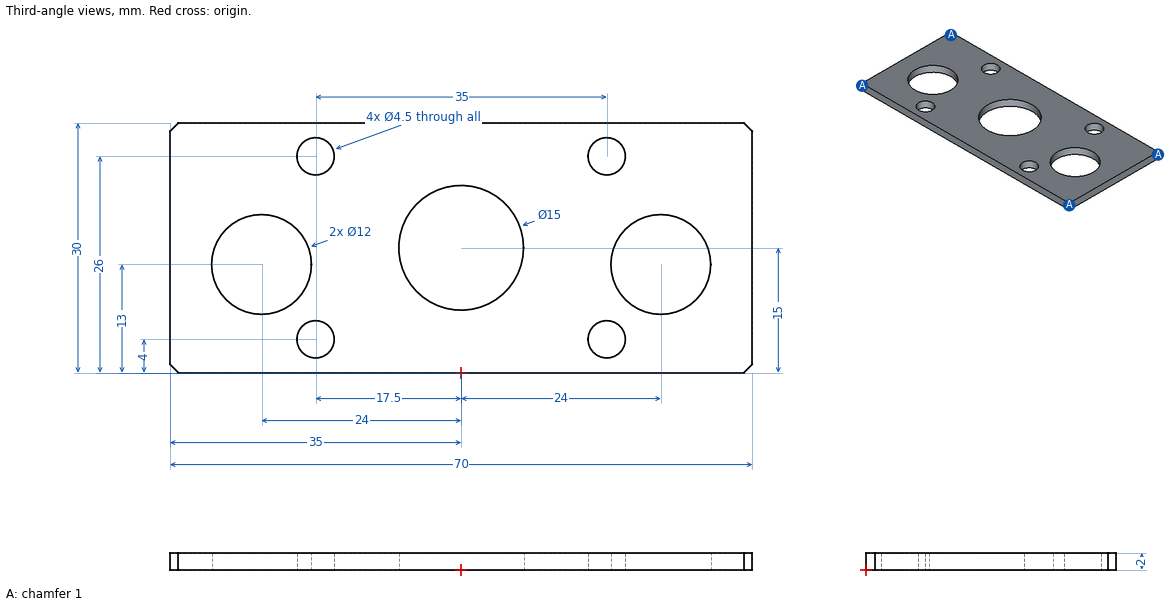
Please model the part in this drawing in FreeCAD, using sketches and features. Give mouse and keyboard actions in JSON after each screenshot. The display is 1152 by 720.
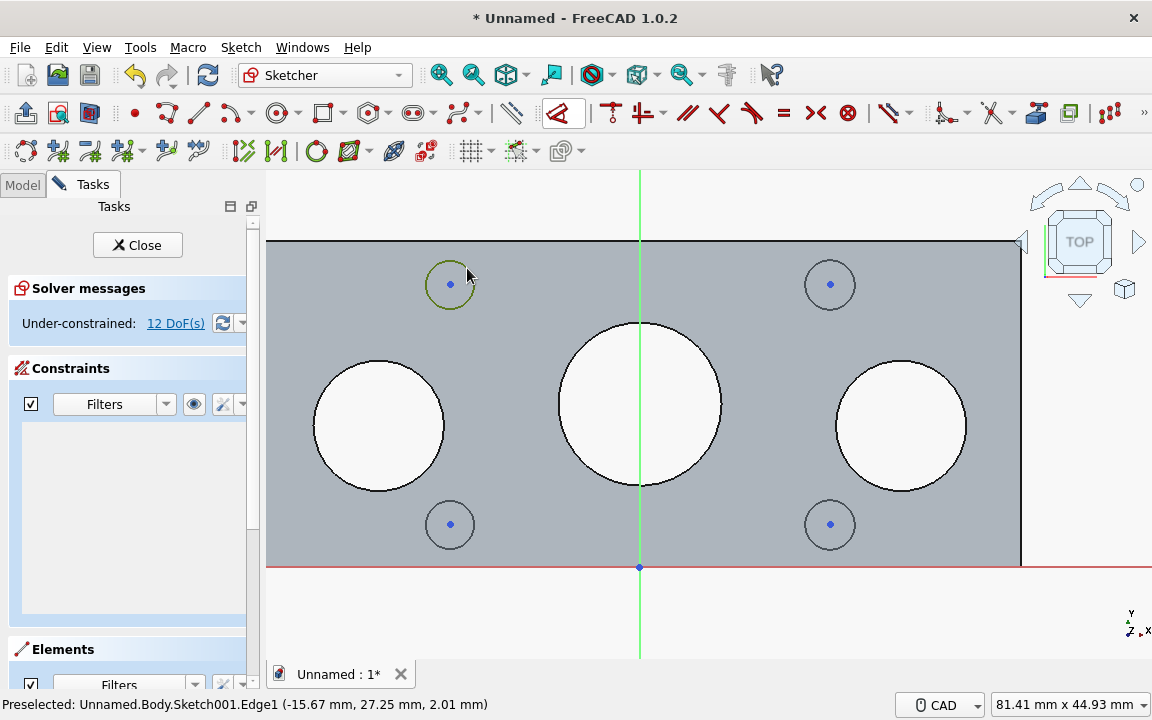
{"action": "left_click", "coordinate": [847, 267]}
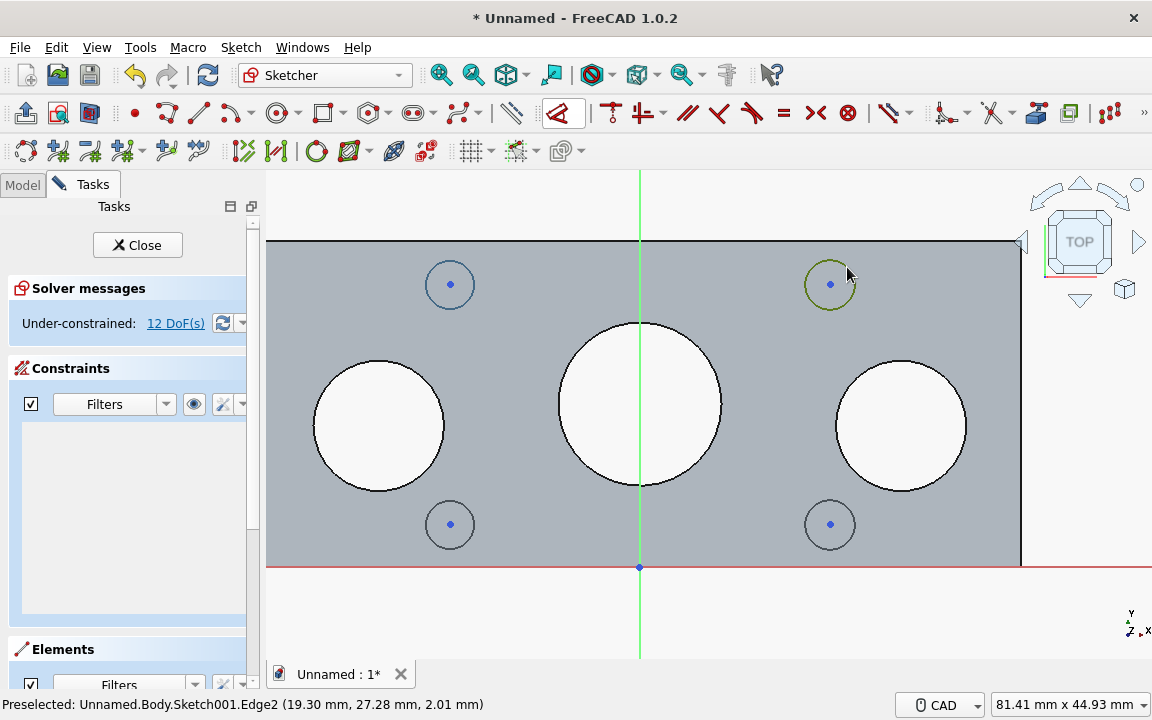
{"action": "left_click", "coordinate": [467, 508]}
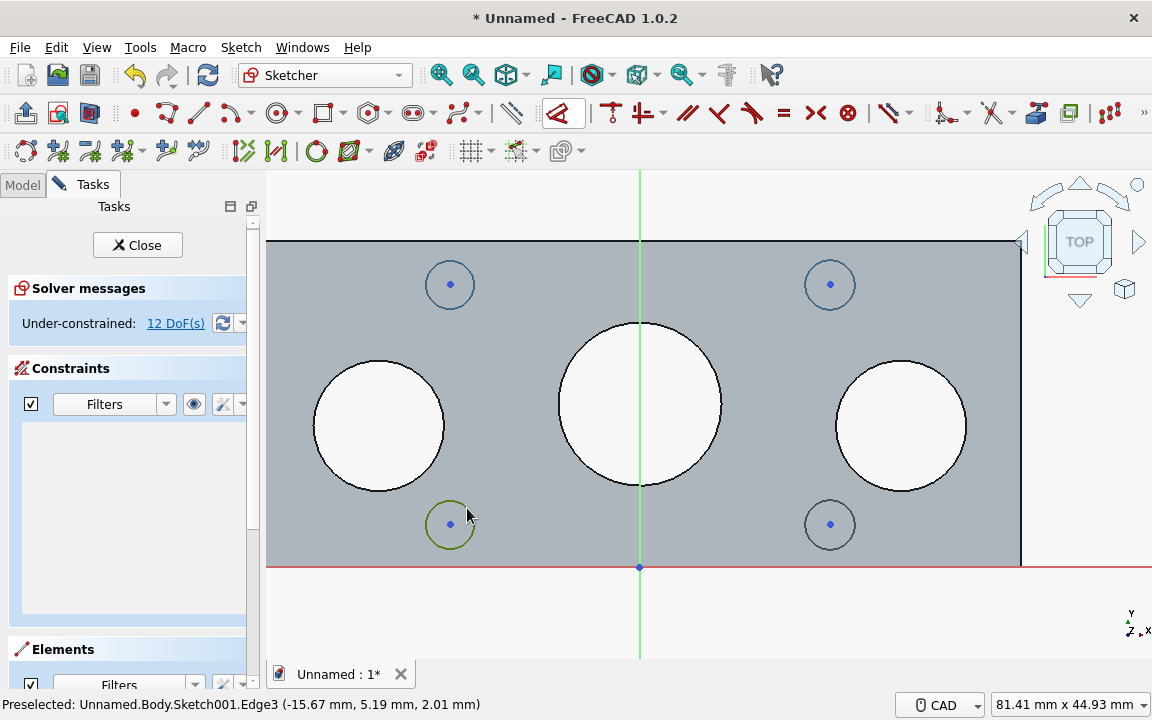
{"action": "left_click", "coordinate": [847, 507]}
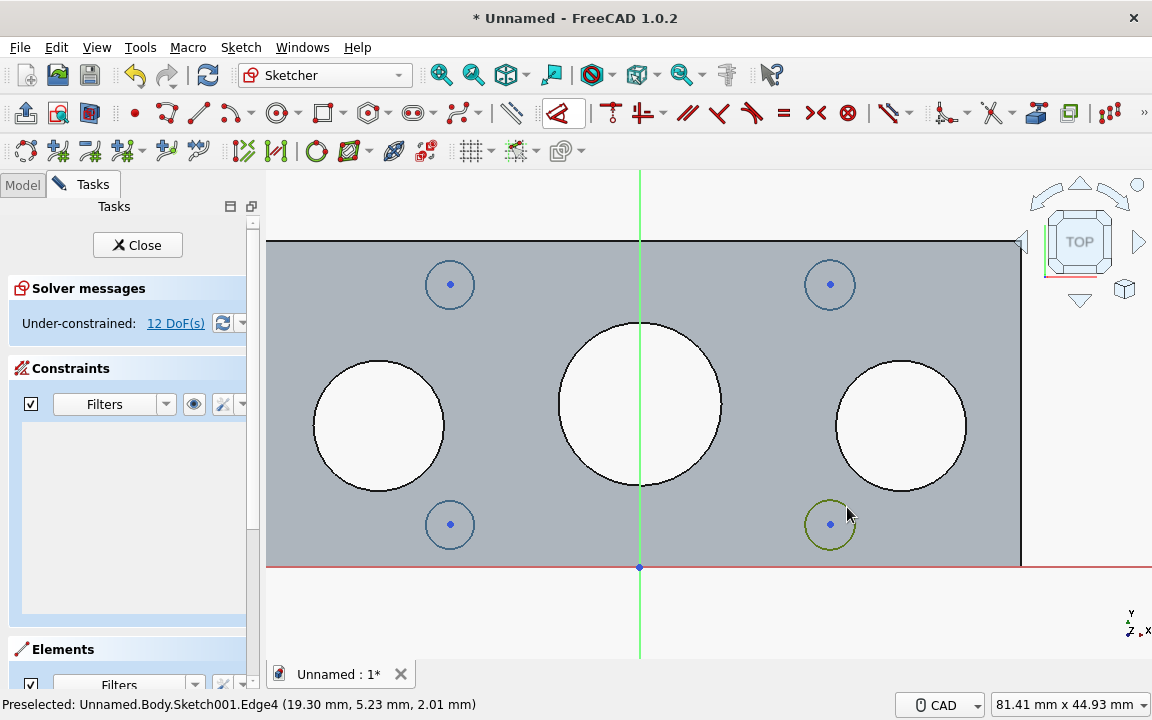
{"action": "left_click", "coordinate": [784, 114]}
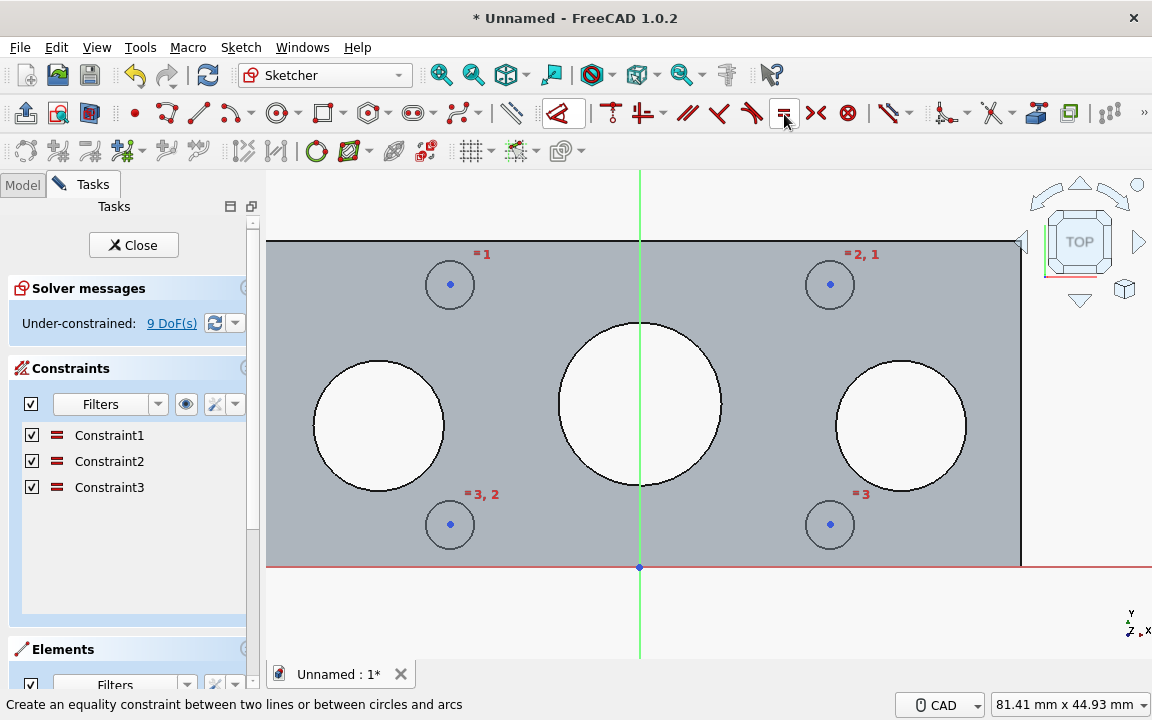
{"action": "left_click", "coordinate": [450, 285]}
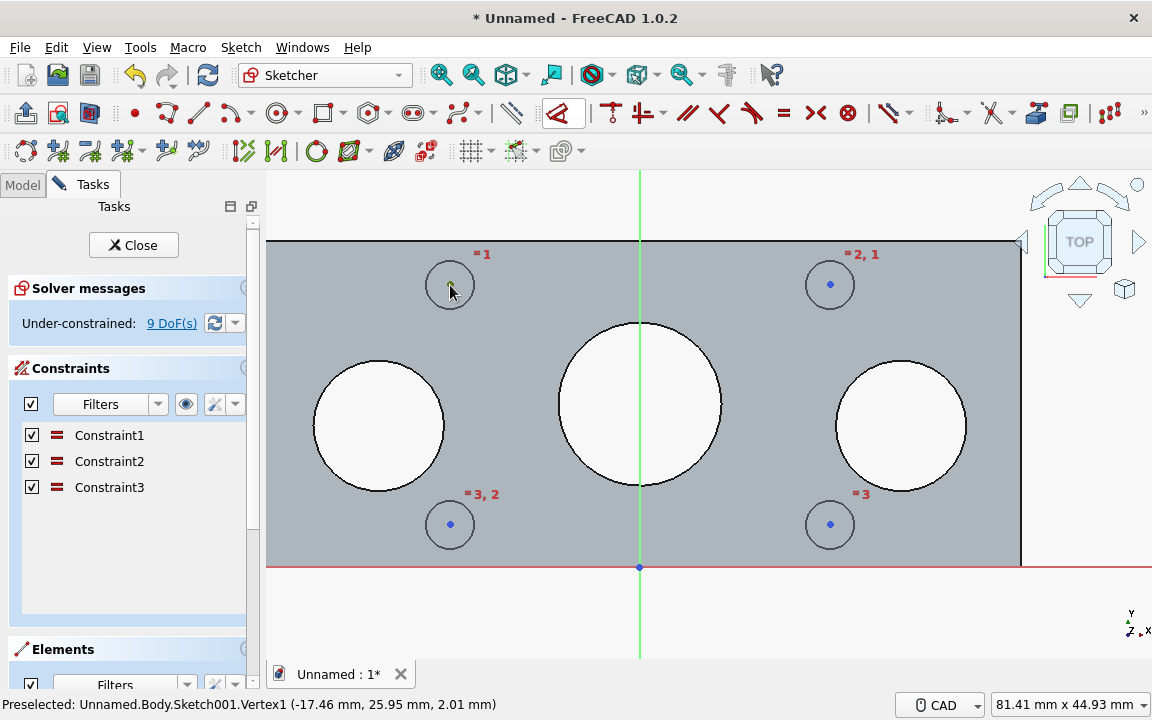
{"action": "left_click", "coordinate": [830, 285]}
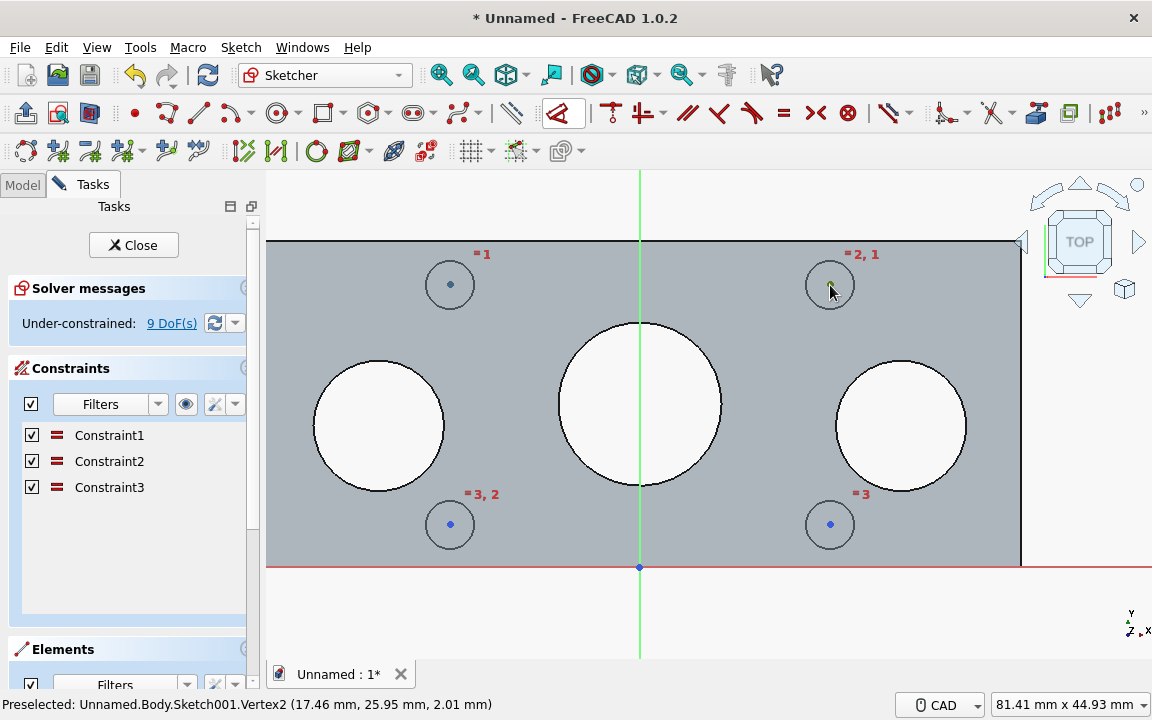
{"action": "left_click", "coordinate": [666, 114]}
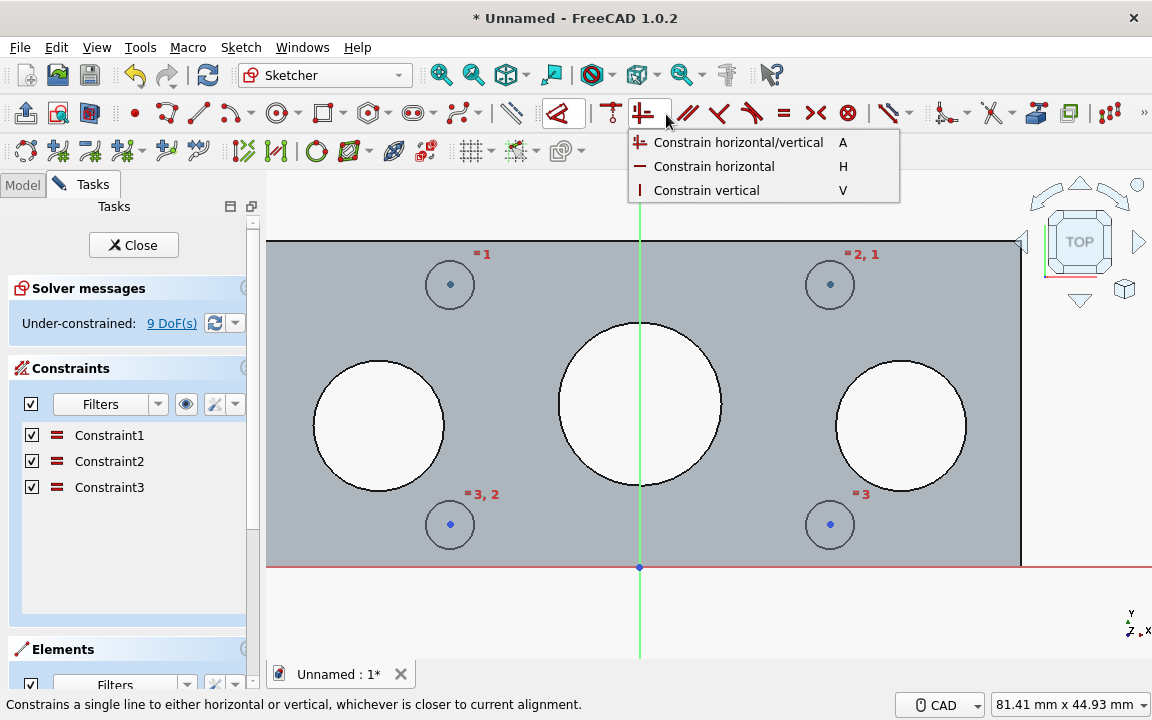
{"action": "left_click", "coordinate": [764, 166]}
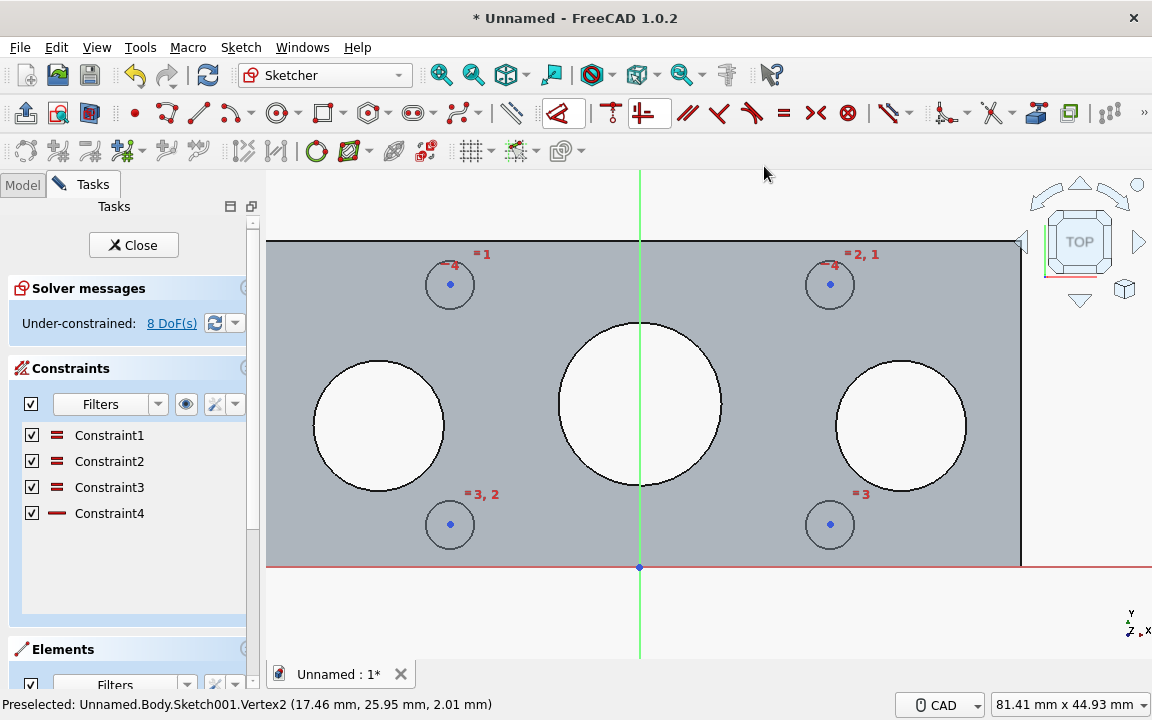
{"action": "left_click", "coordinate": [450, 285]}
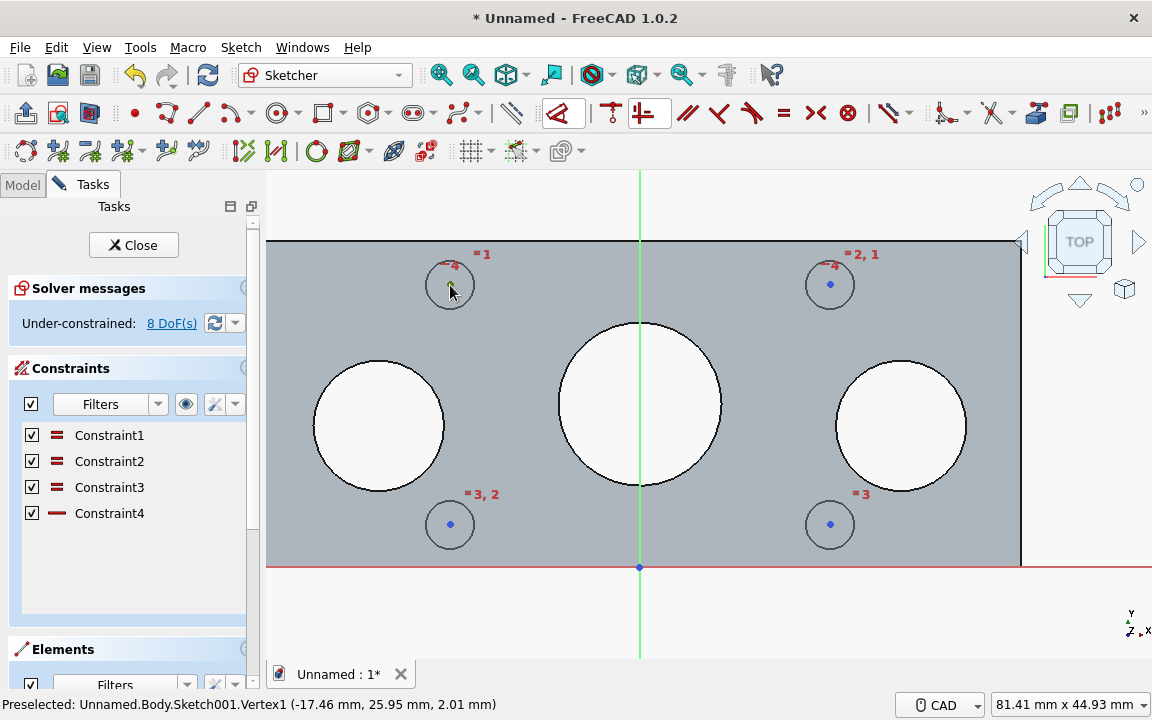
{"action": "left_click", "coordinate": [450, 525]}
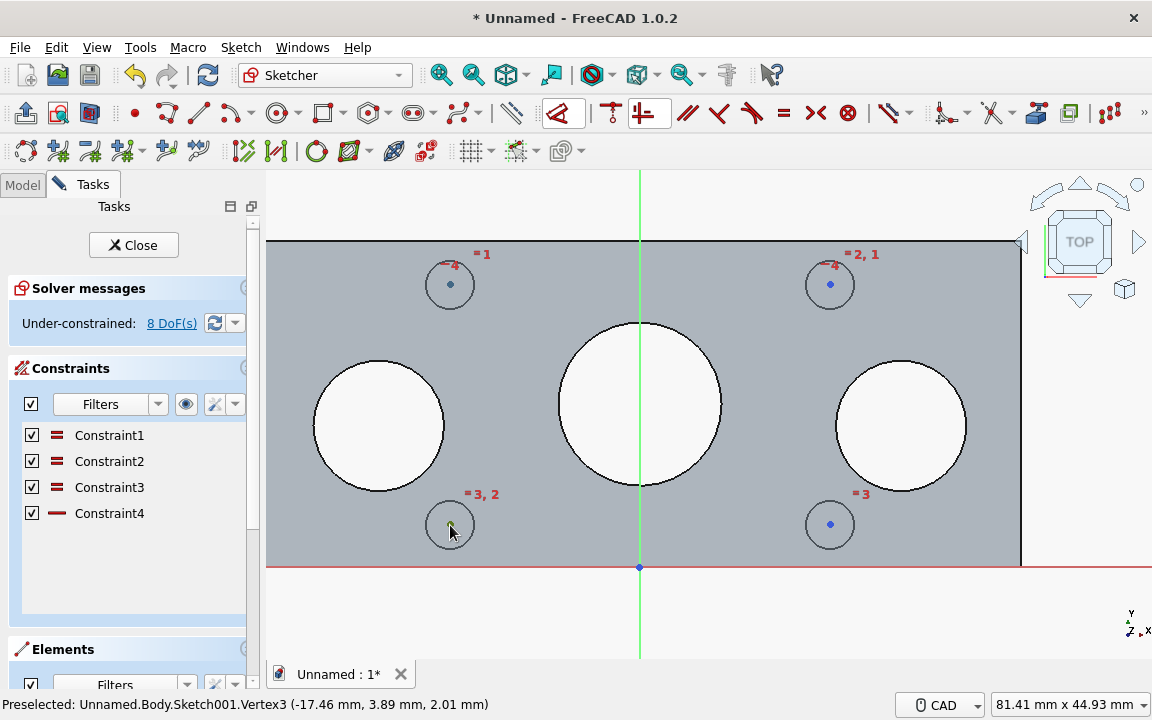
{"action": "key", "text": "v"}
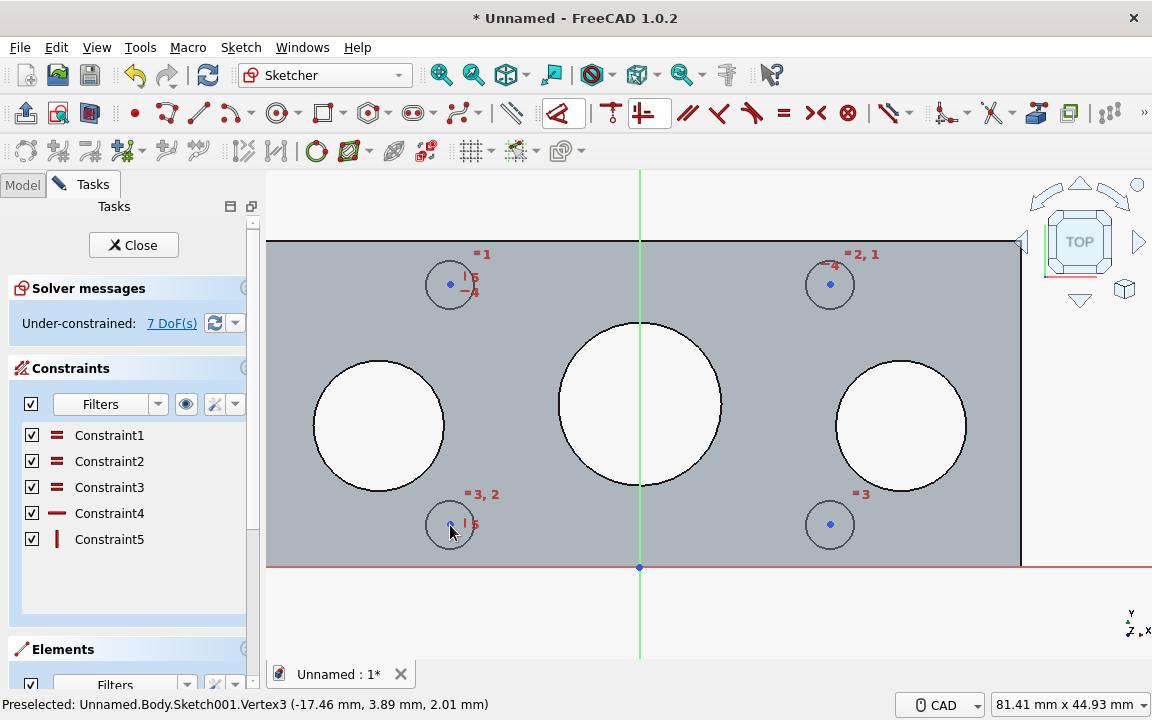
{"action": "left_click", "coordinate": [830, 285]}